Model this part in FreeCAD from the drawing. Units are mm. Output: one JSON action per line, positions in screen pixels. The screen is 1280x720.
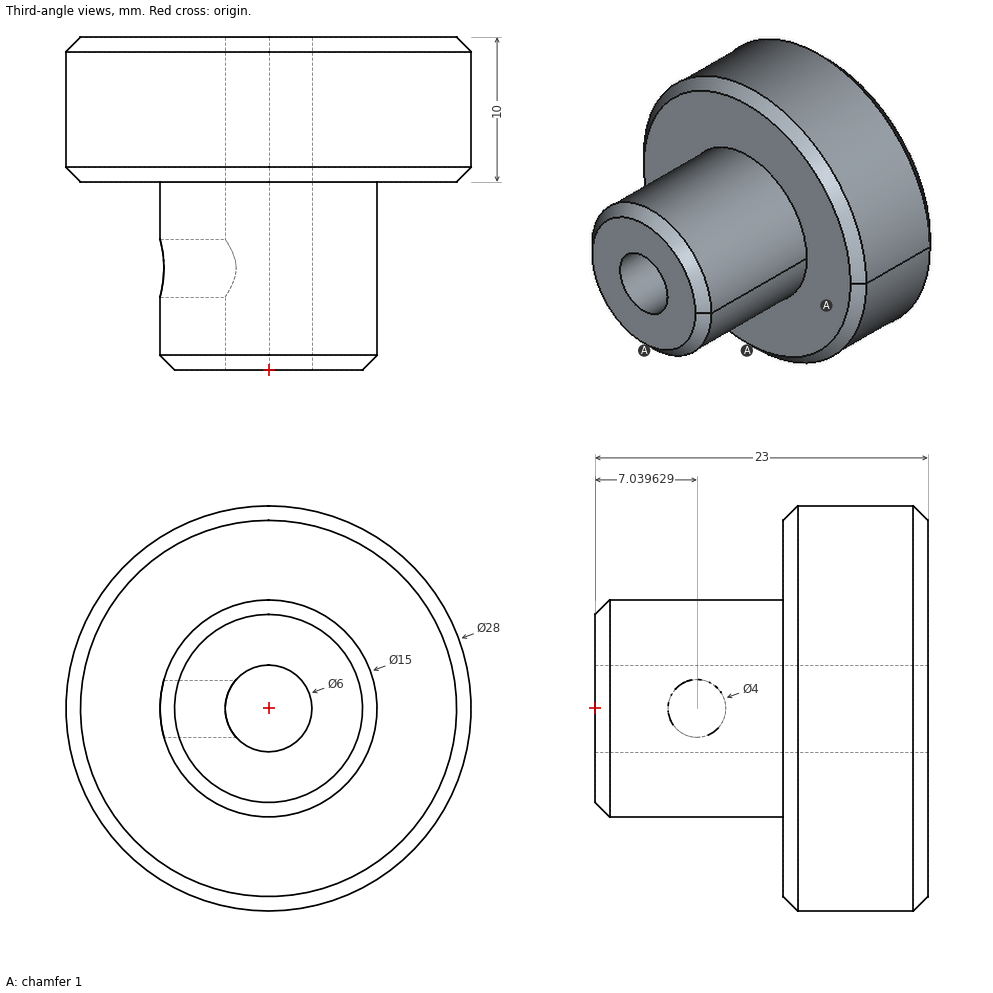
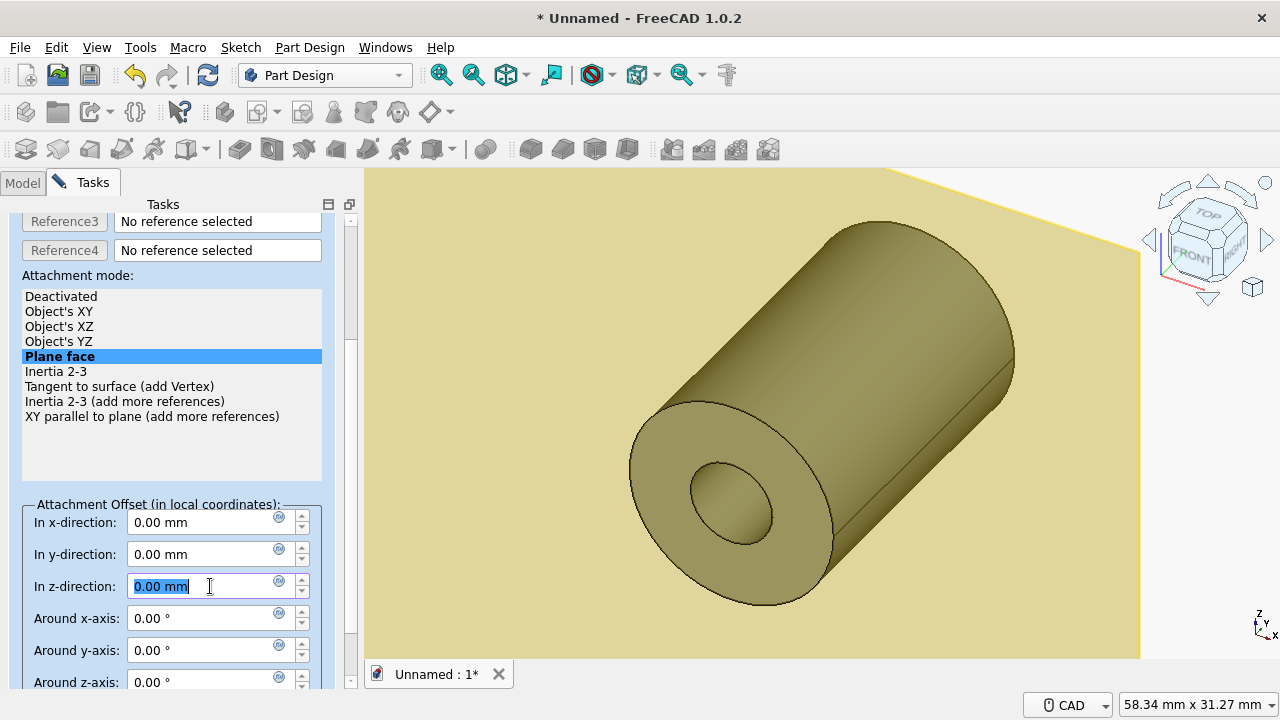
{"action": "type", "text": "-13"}
{"action": "key", "text": "Tab"}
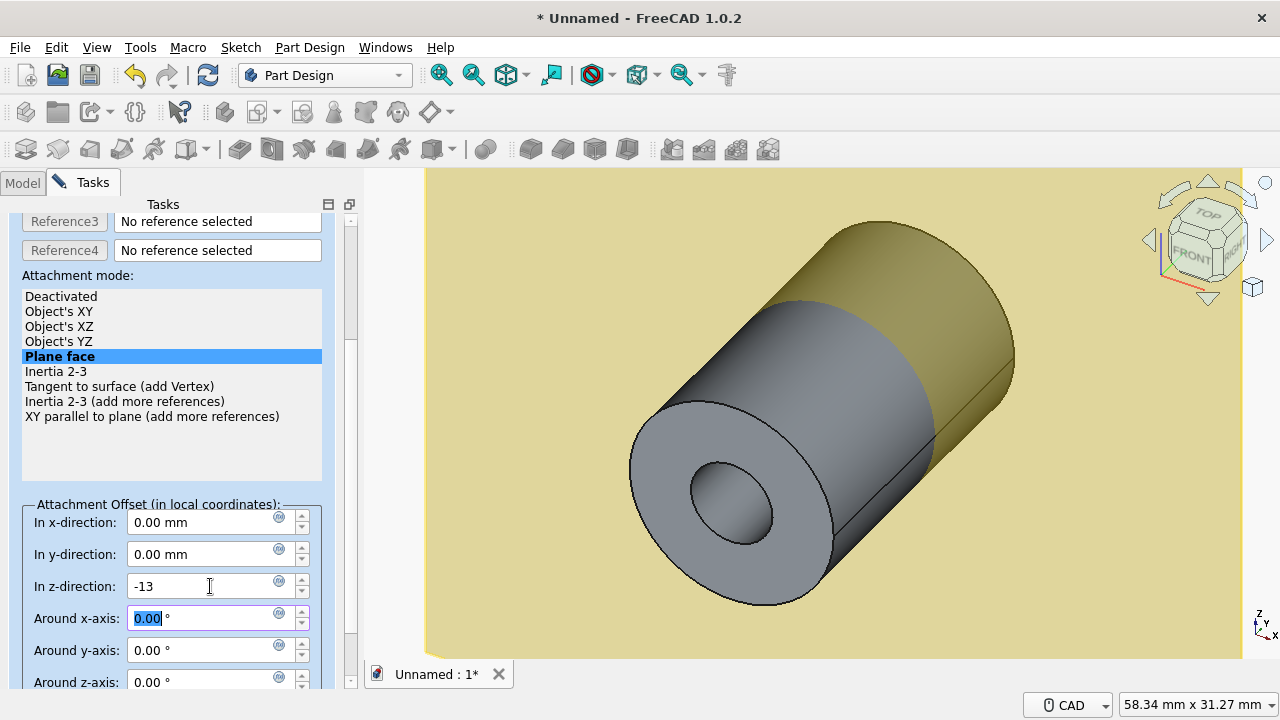
{"action": "scroll", "coordinate": [351, 451], "scroll_direction": "up", "scroll_amount": 4}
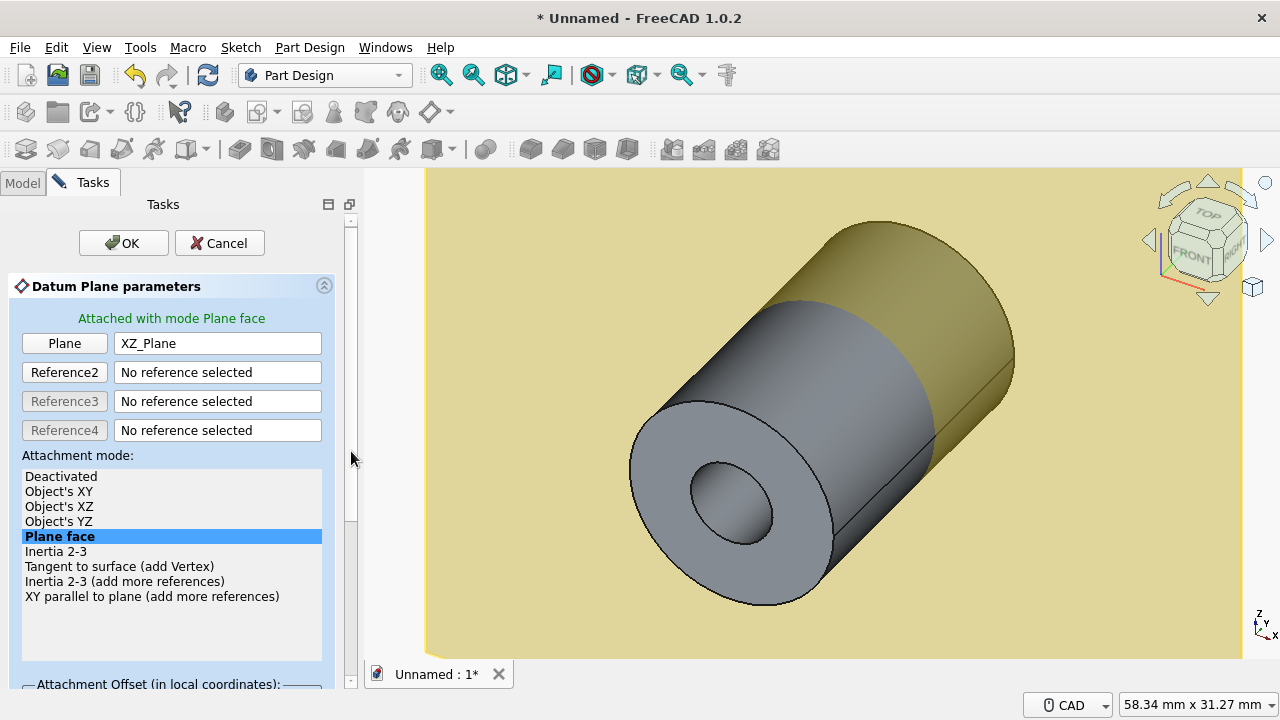
{"action": "left_click", "coordinate": [124, 243]}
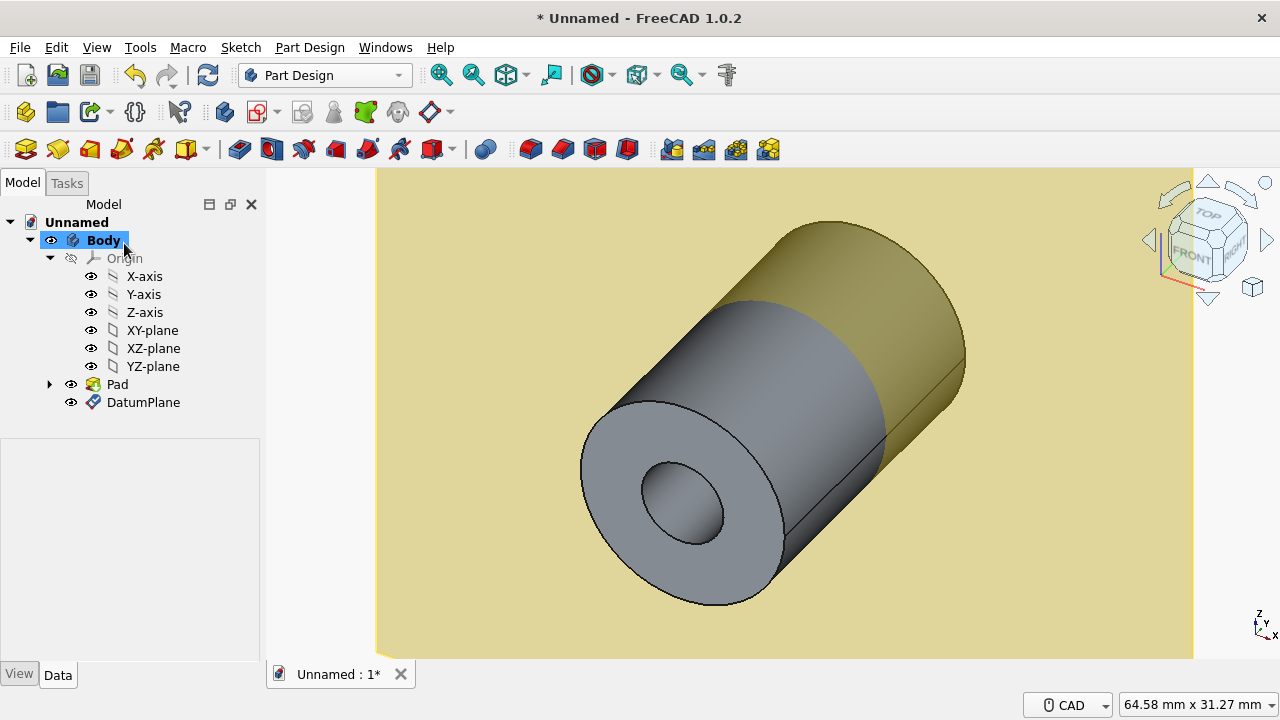
{"action": "left_click", "coordinate": [116, 402]}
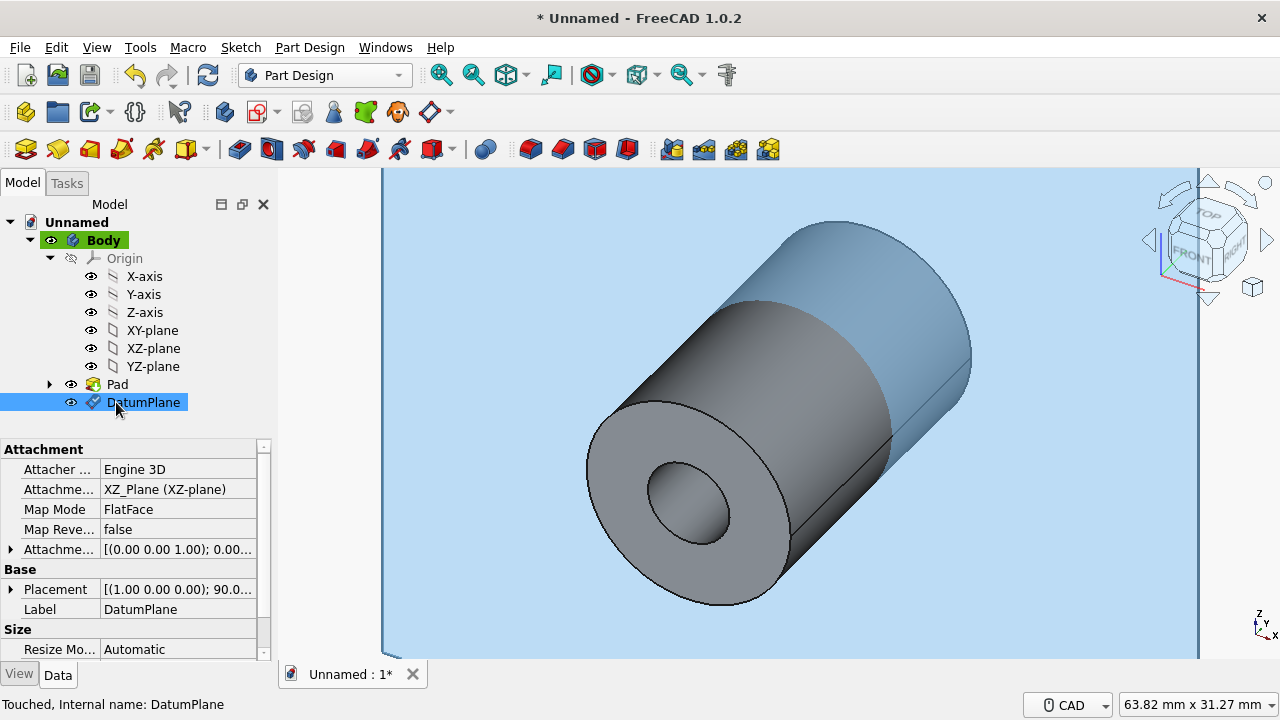
{"action": "left_click", "coordinate": [258, 112]}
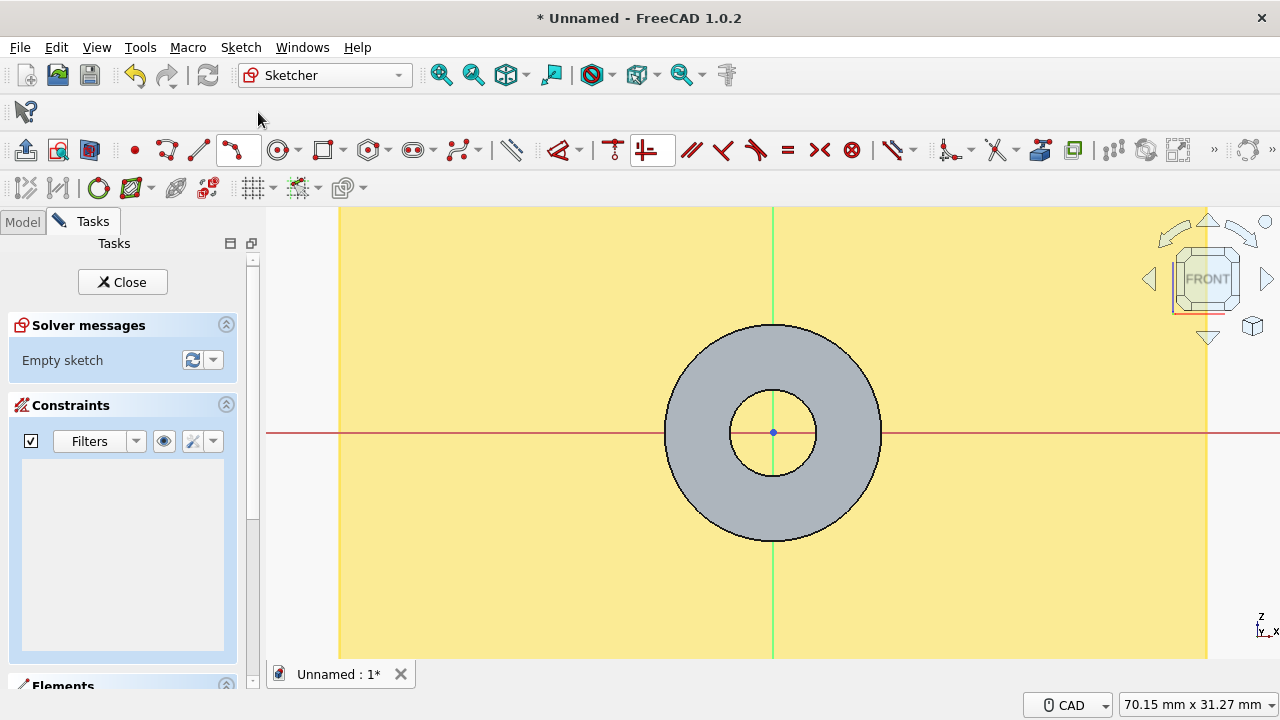
{"action": "left_click", "coordinate": [90, 150]}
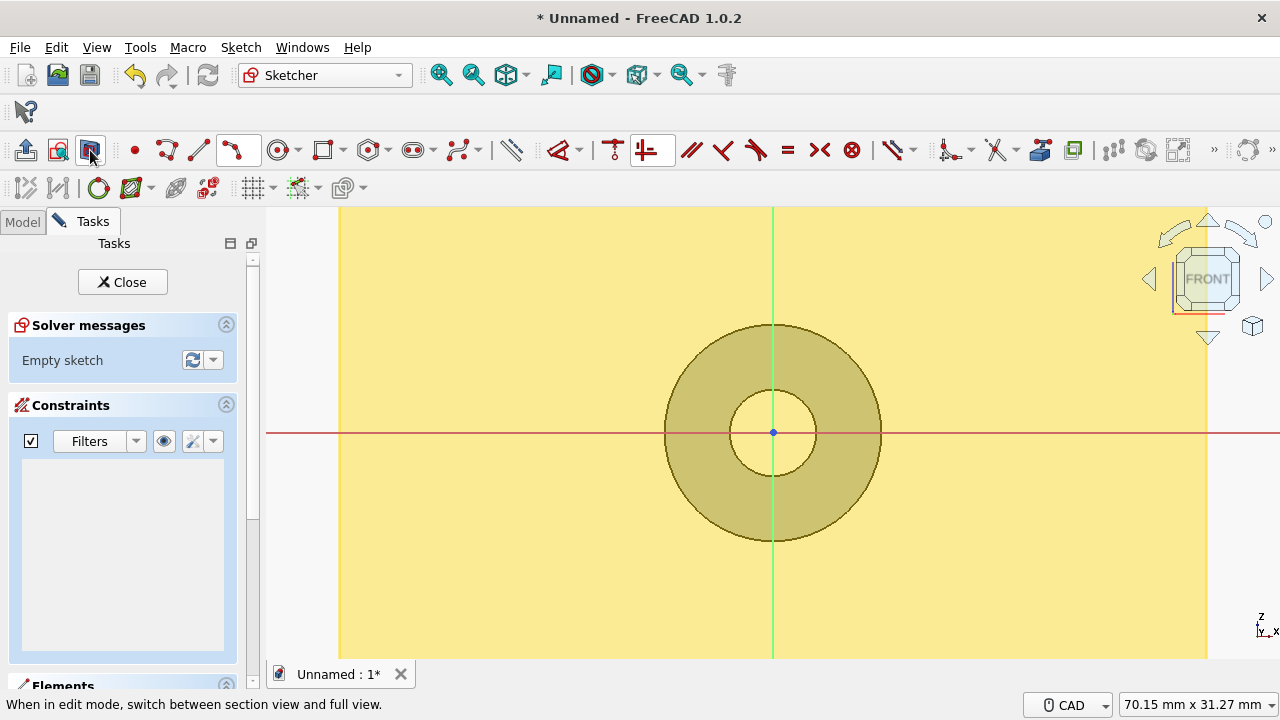
{"action": "scroll", "coordinate": [565, 433], "scroll_direction": "down", "scroll_amount": 2}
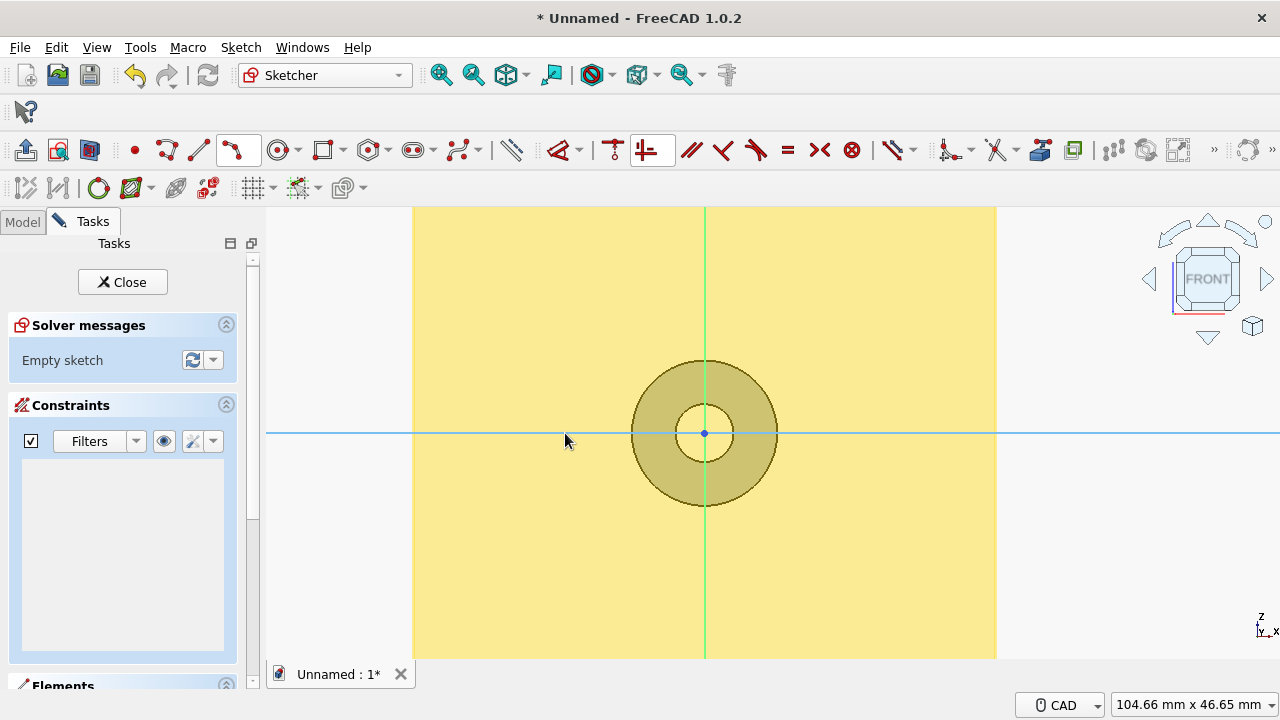
{"action": "left_click", "coordinate": [278, 150]}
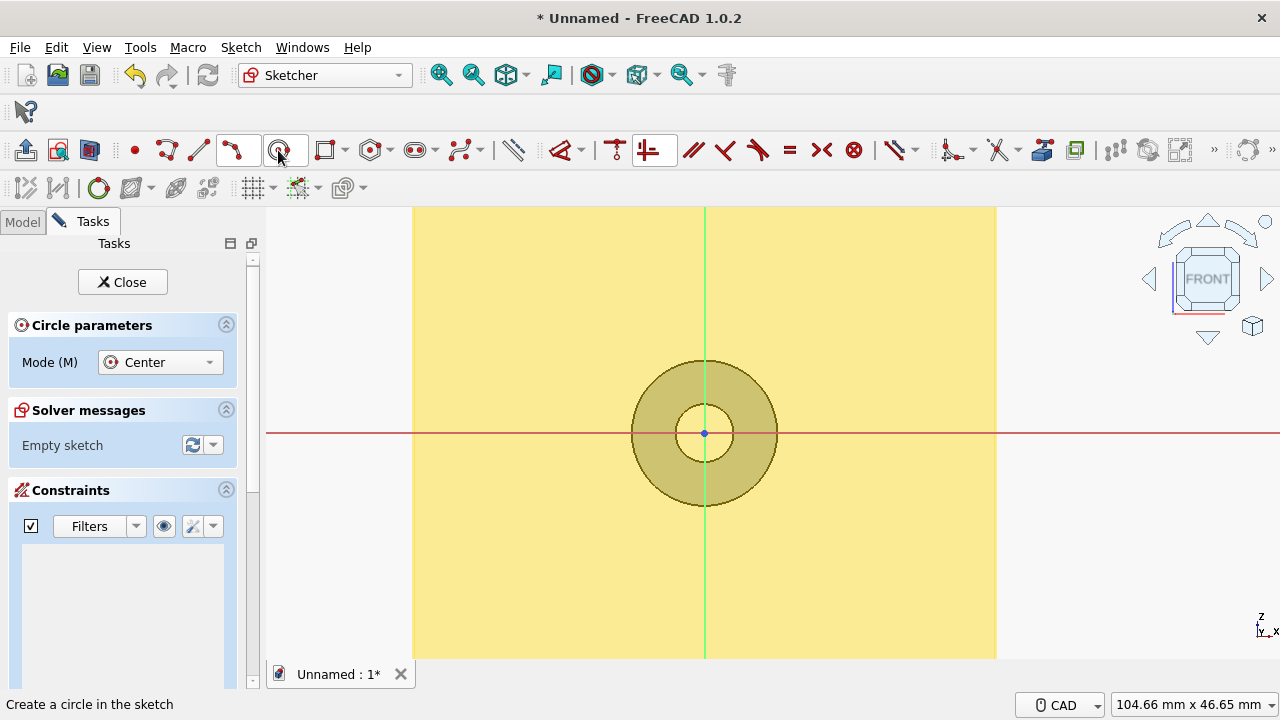
{"action": "left_click", "coordinate": [705, 433]}
{"action": "mouse_move", "coordinate": [800, 337]}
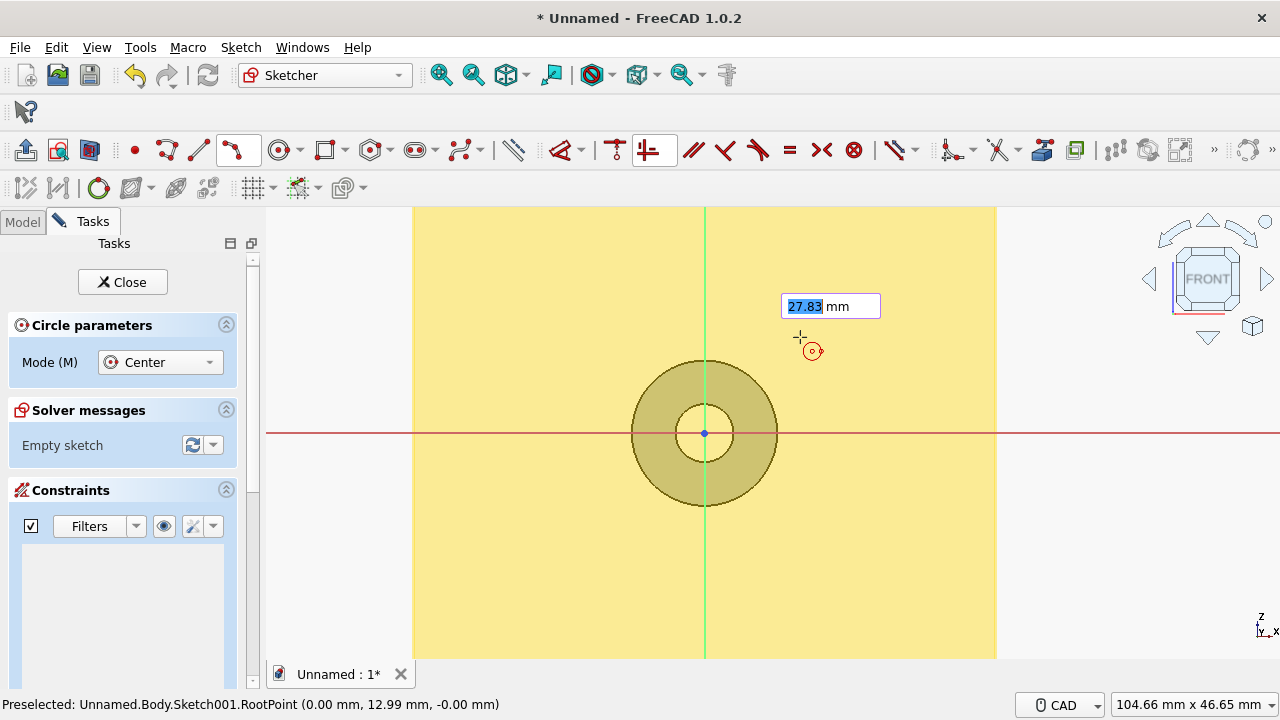
{"action": "type", "text": "28"}
{"action": "key", "text": "Return"}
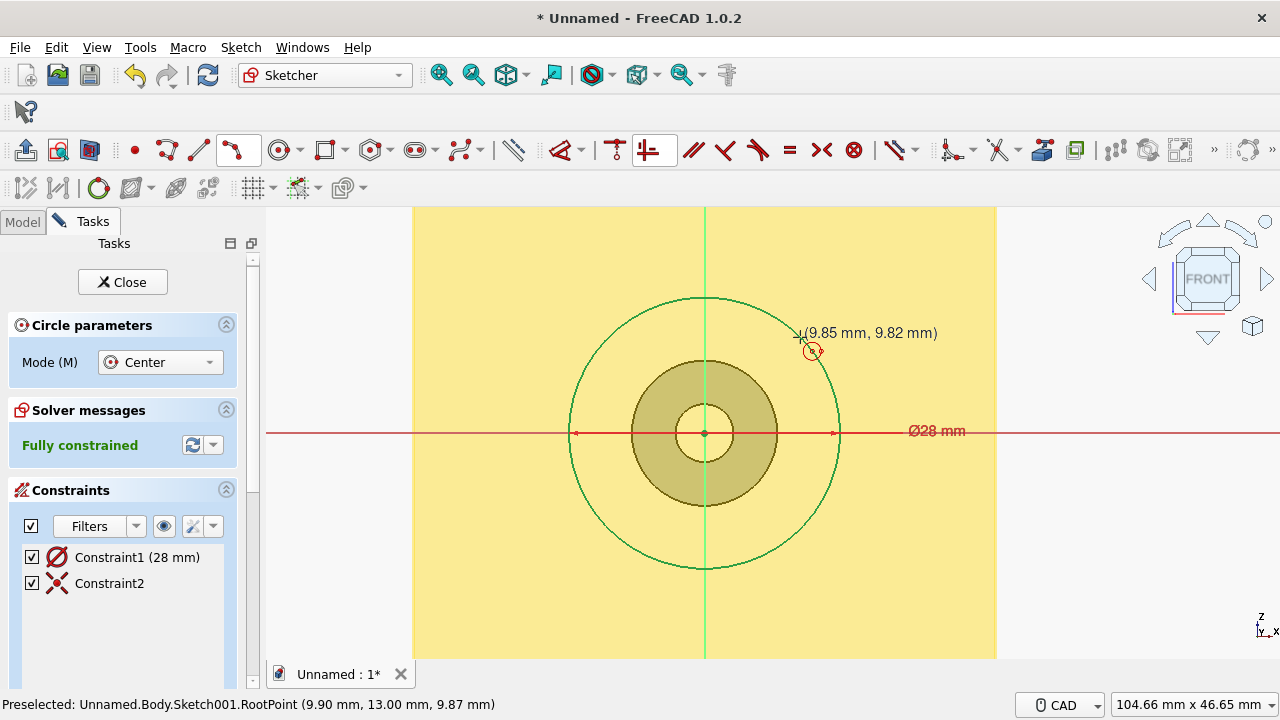
{"action": "left_click", "coordinate": [705, 433]}
{"action": "mouse_move", "coordinate": [725, 413]}